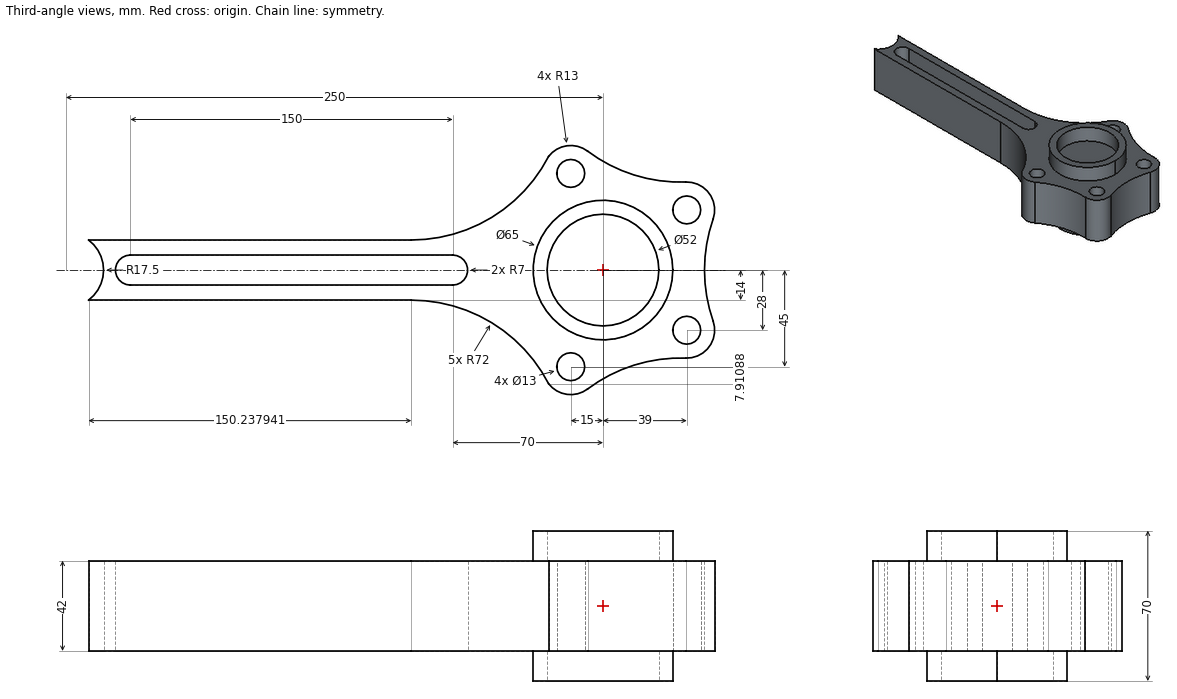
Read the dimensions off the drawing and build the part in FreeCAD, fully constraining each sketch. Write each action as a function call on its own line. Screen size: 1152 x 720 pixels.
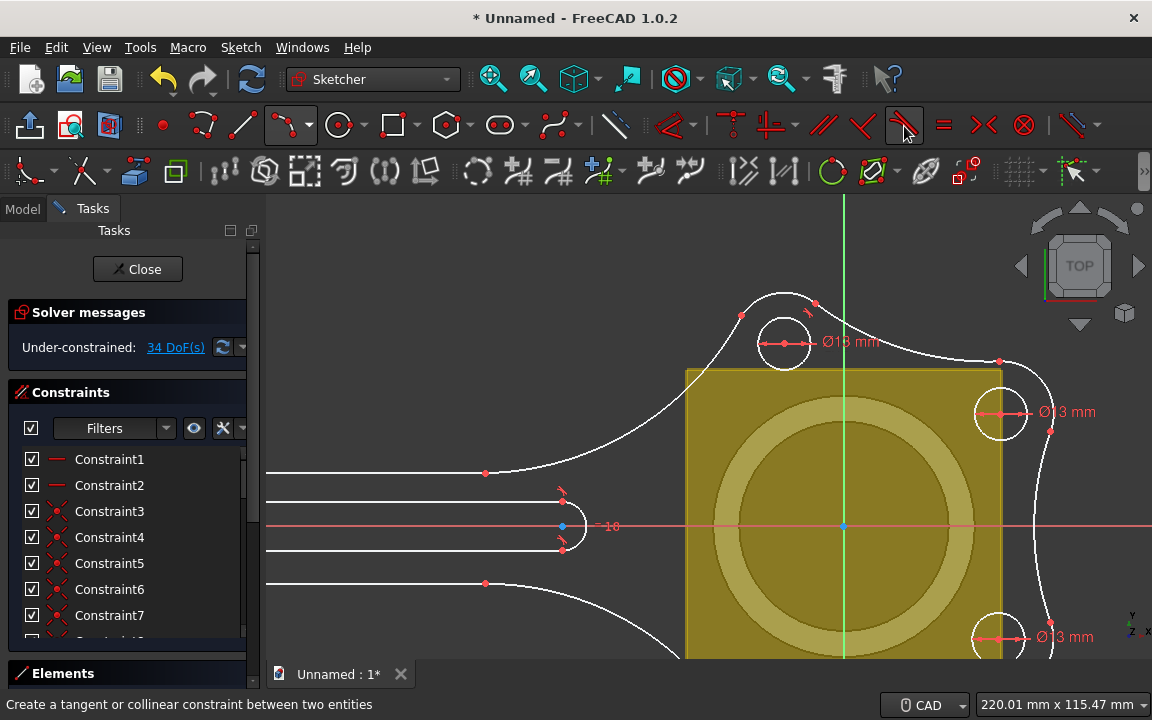
click(866, 334)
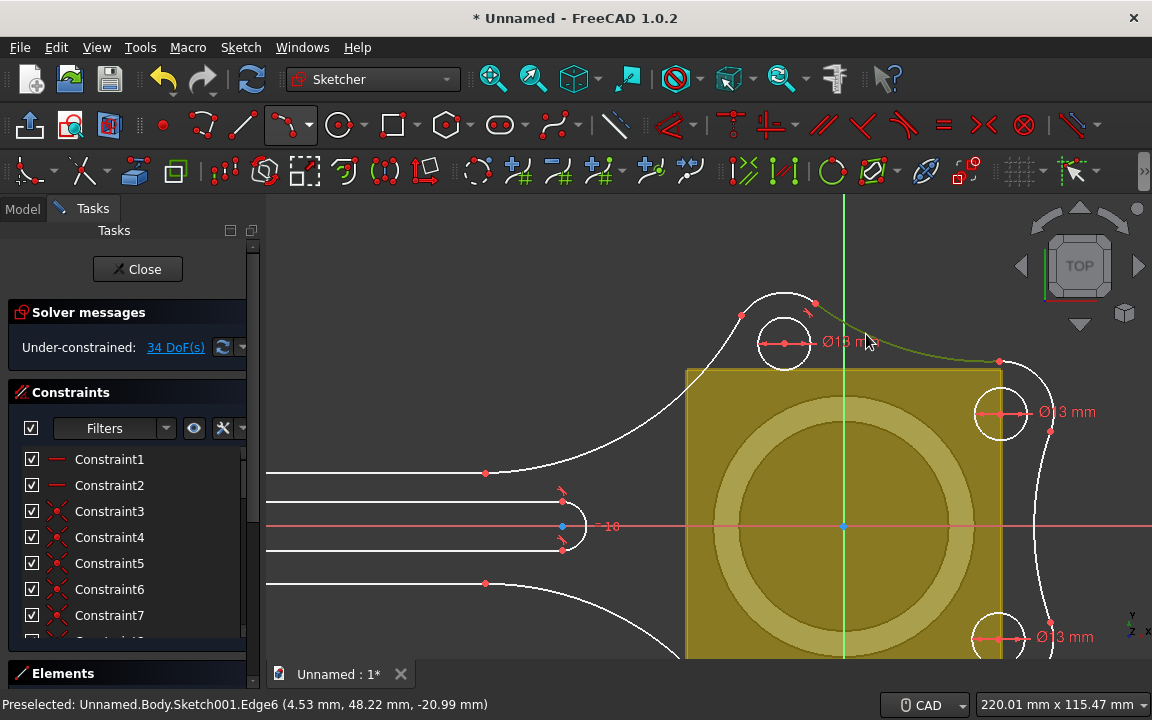
scroll(784, 345, down, 4)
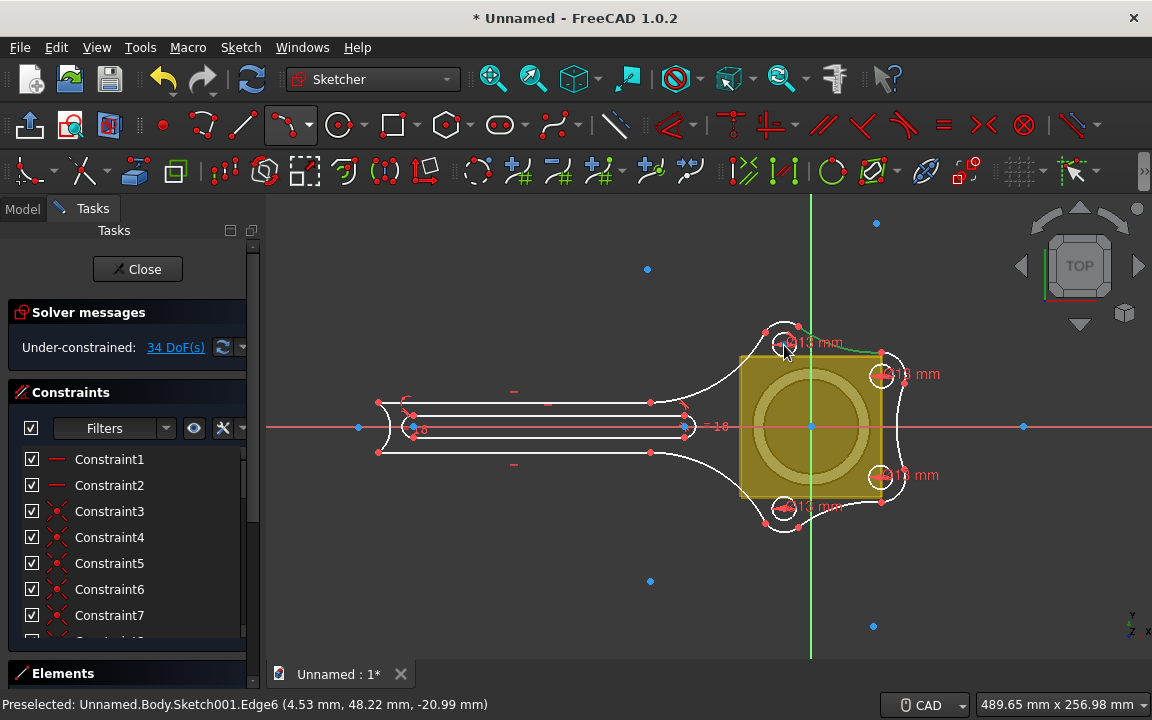
click(894, 356)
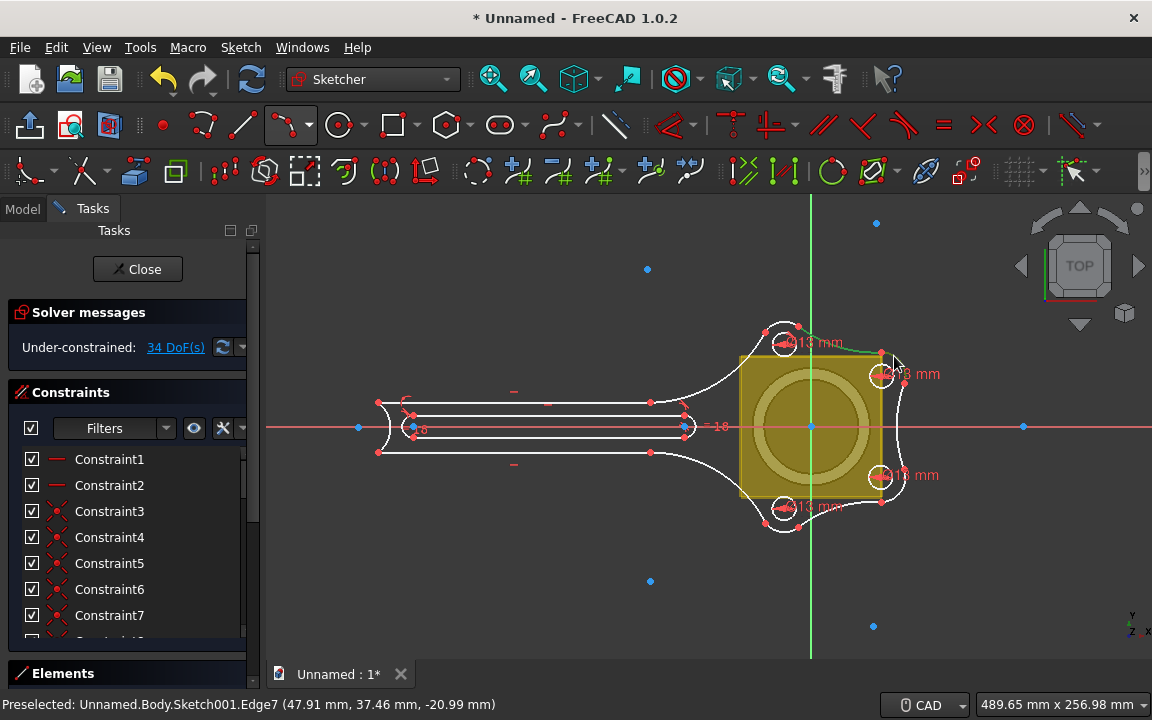
click(904, 126)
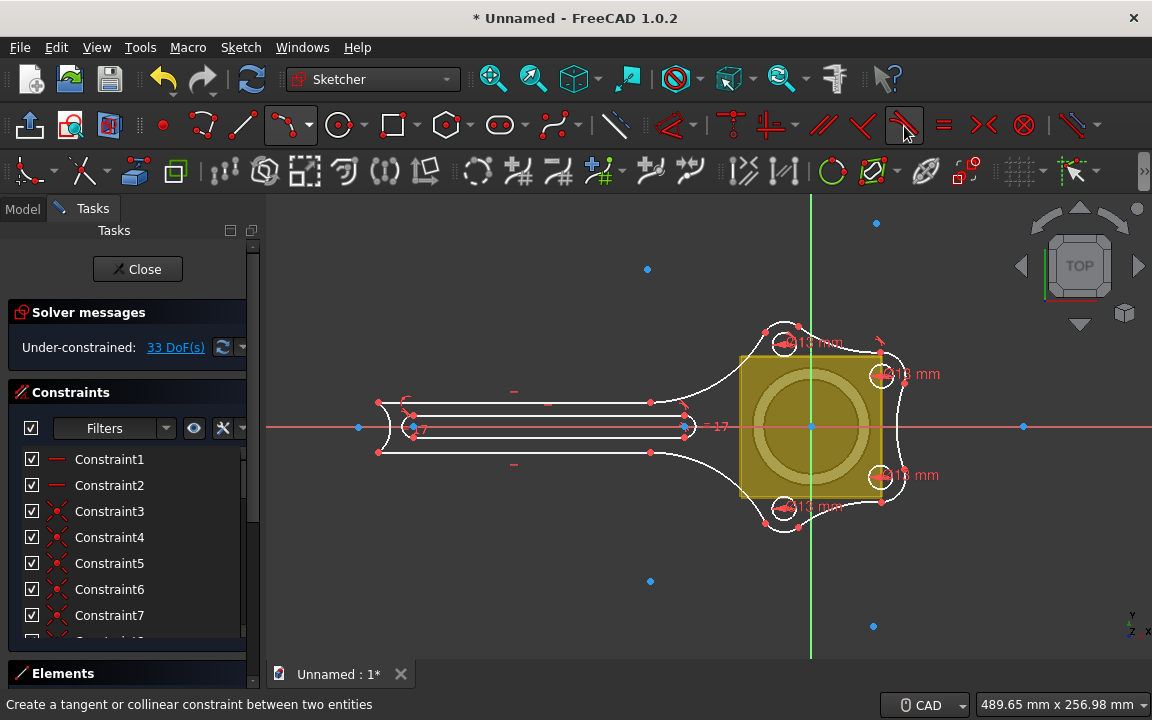
click(905, 370)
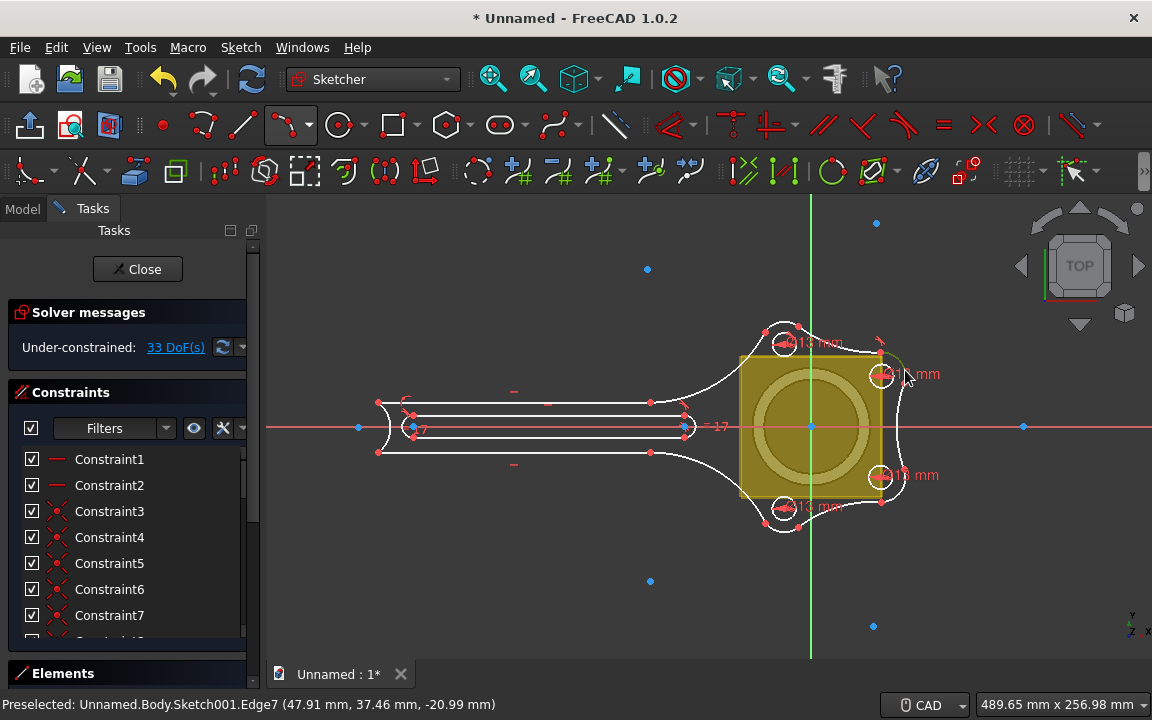
click(898, 409)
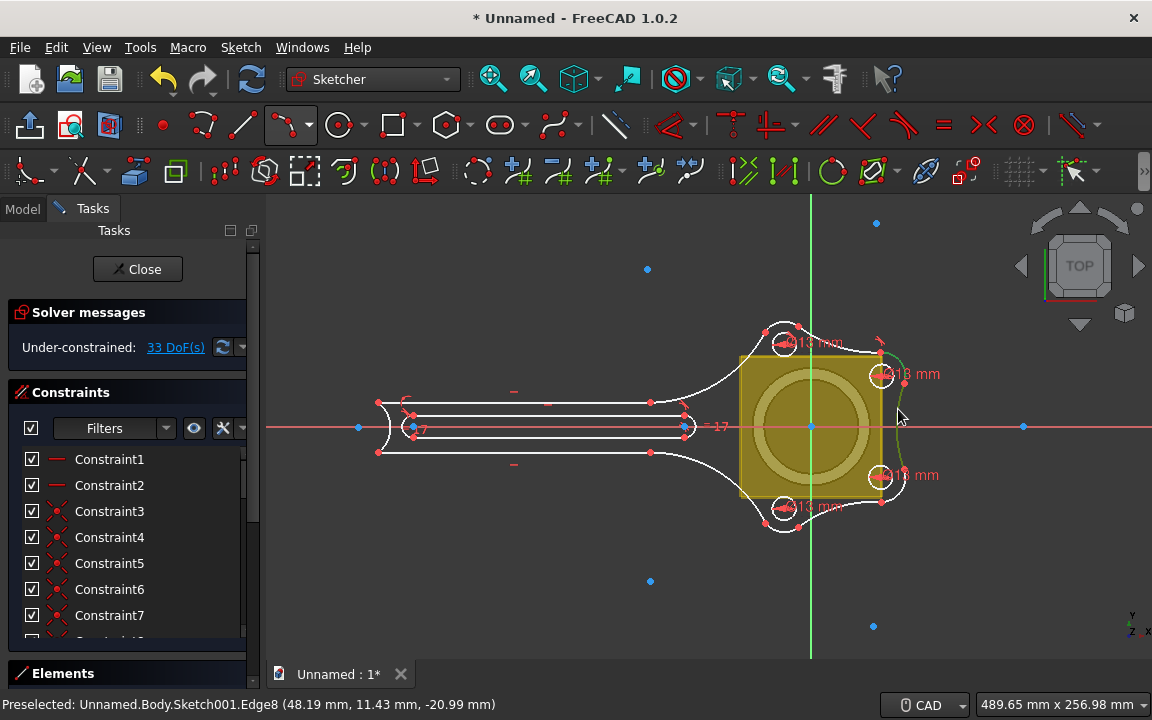
click(904, 126)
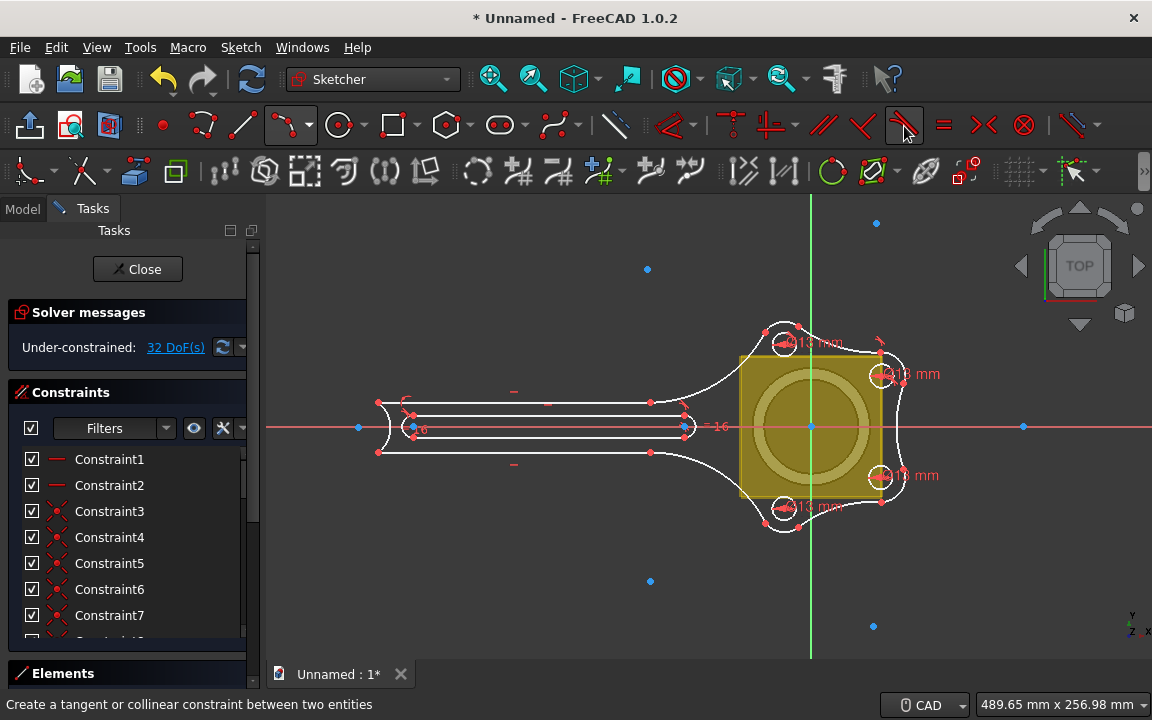
click(898, 409)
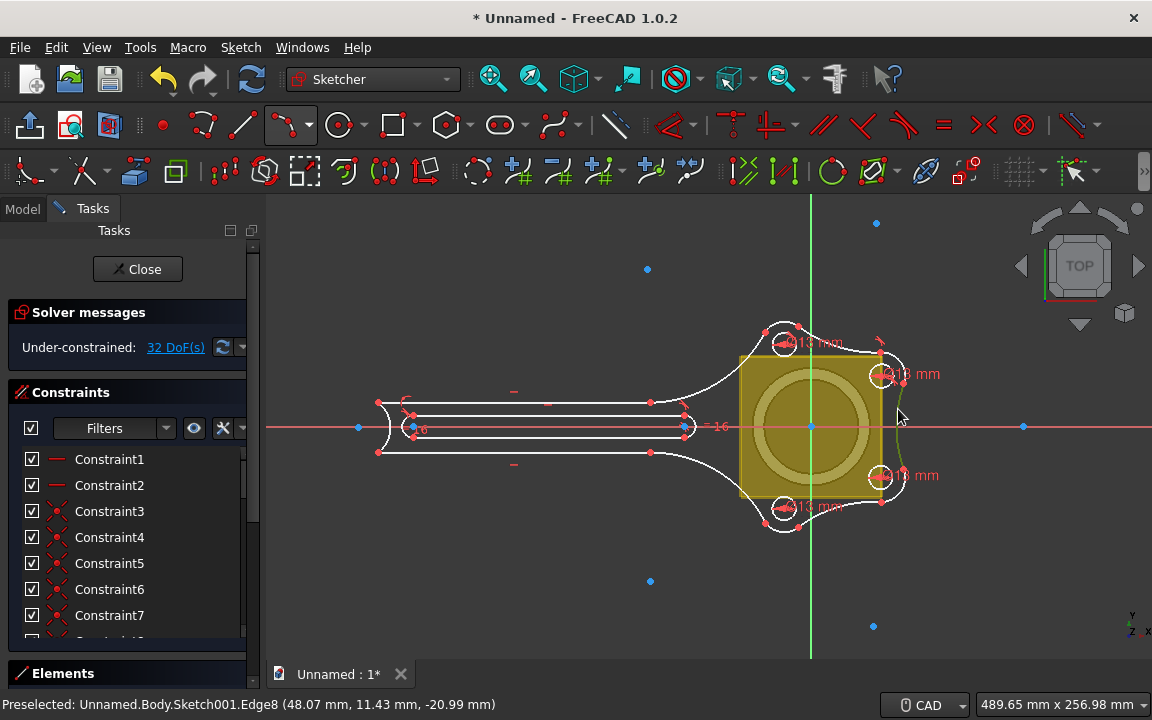
click(894, 498)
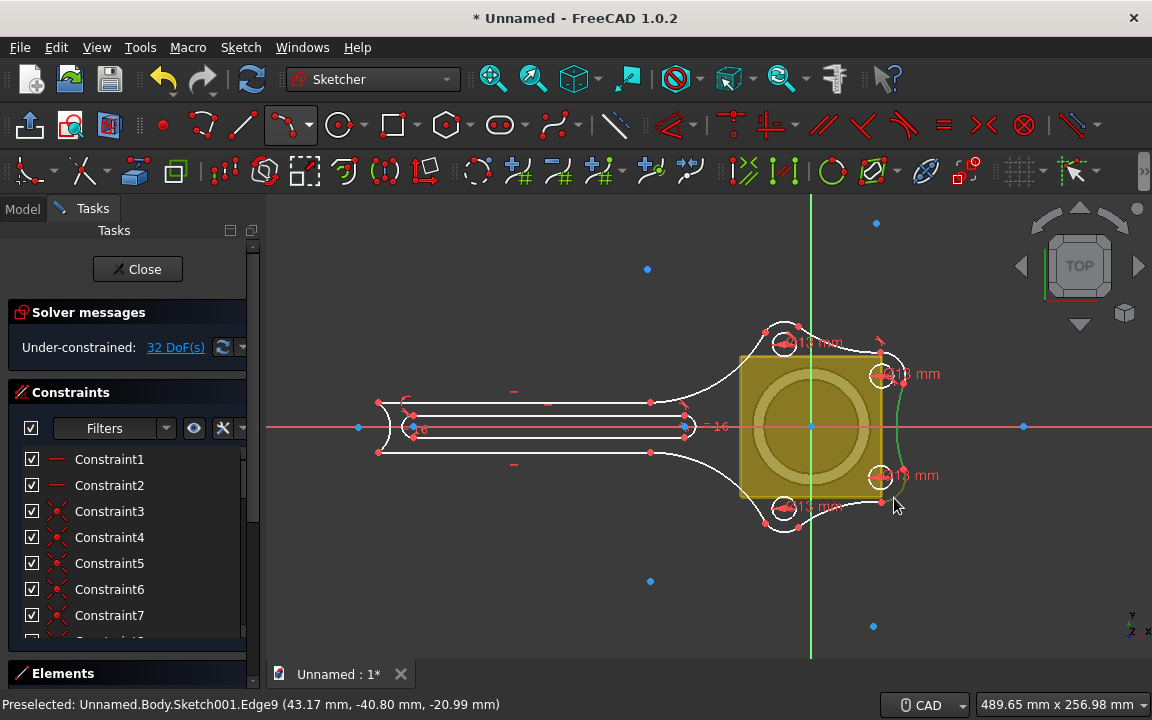
click(904, 126)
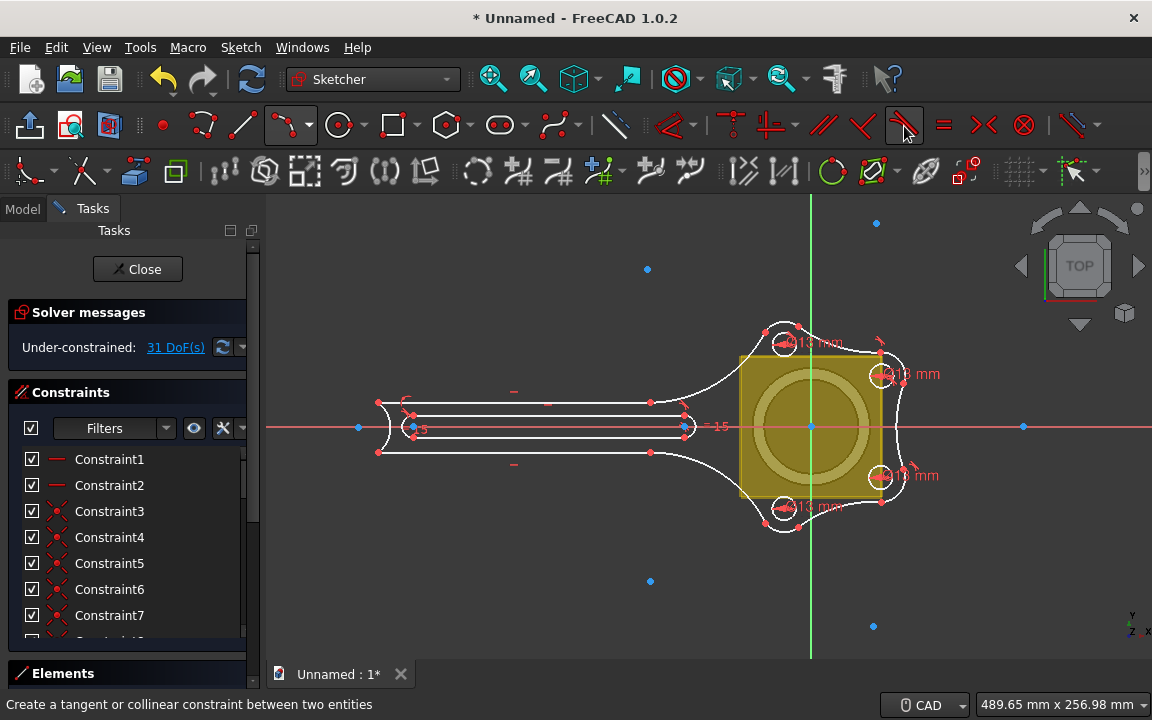
click(894, 498)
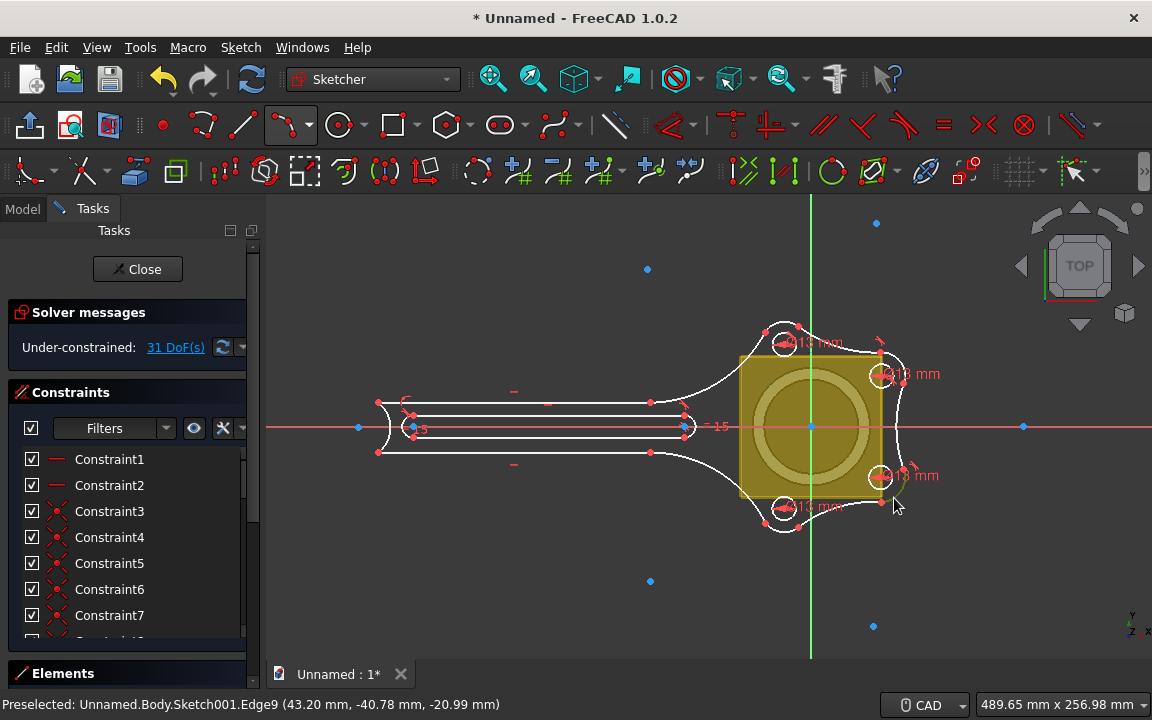
click(855, 503)